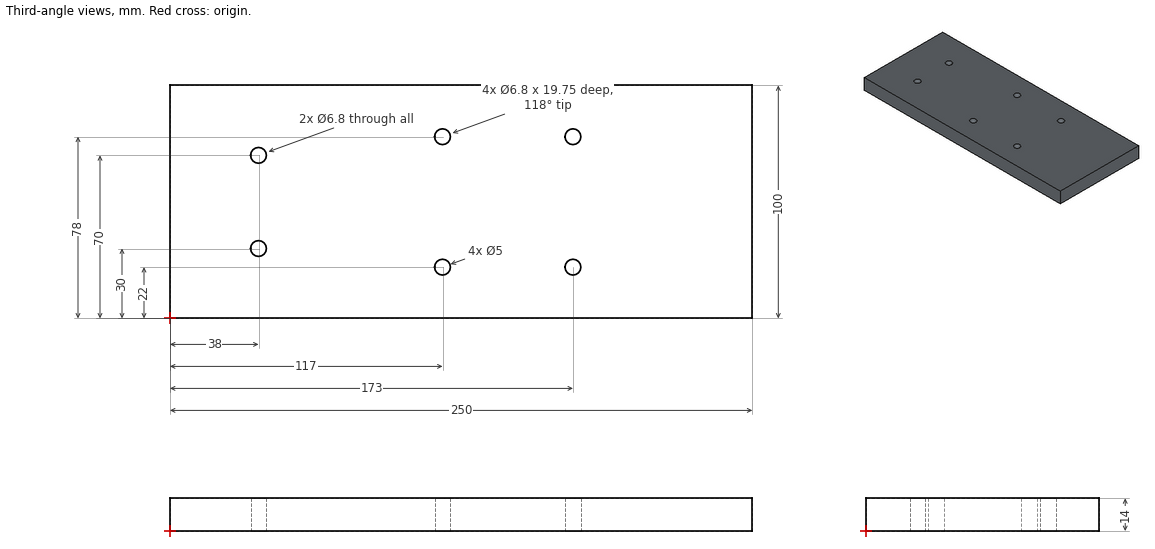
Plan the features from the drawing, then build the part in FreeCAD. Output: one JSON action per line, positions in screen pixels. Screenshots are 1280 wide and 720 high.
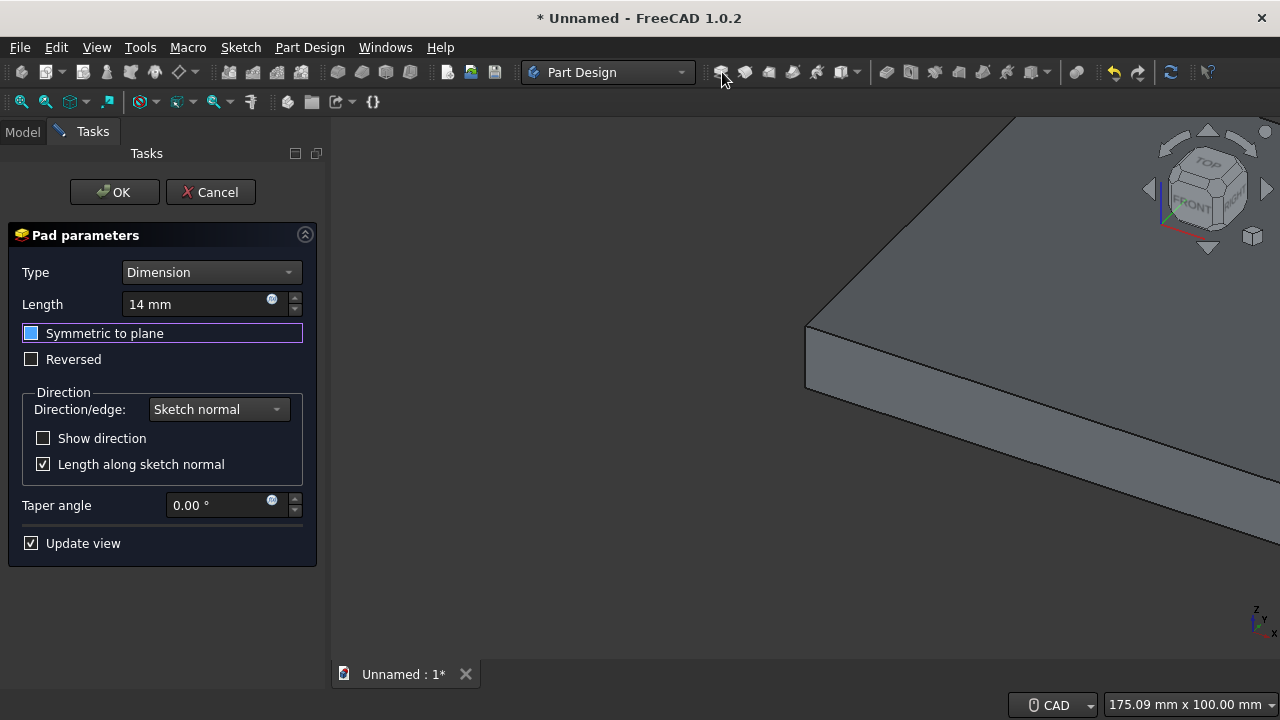
{"action": "left_click", "coordinate": [115, 192]}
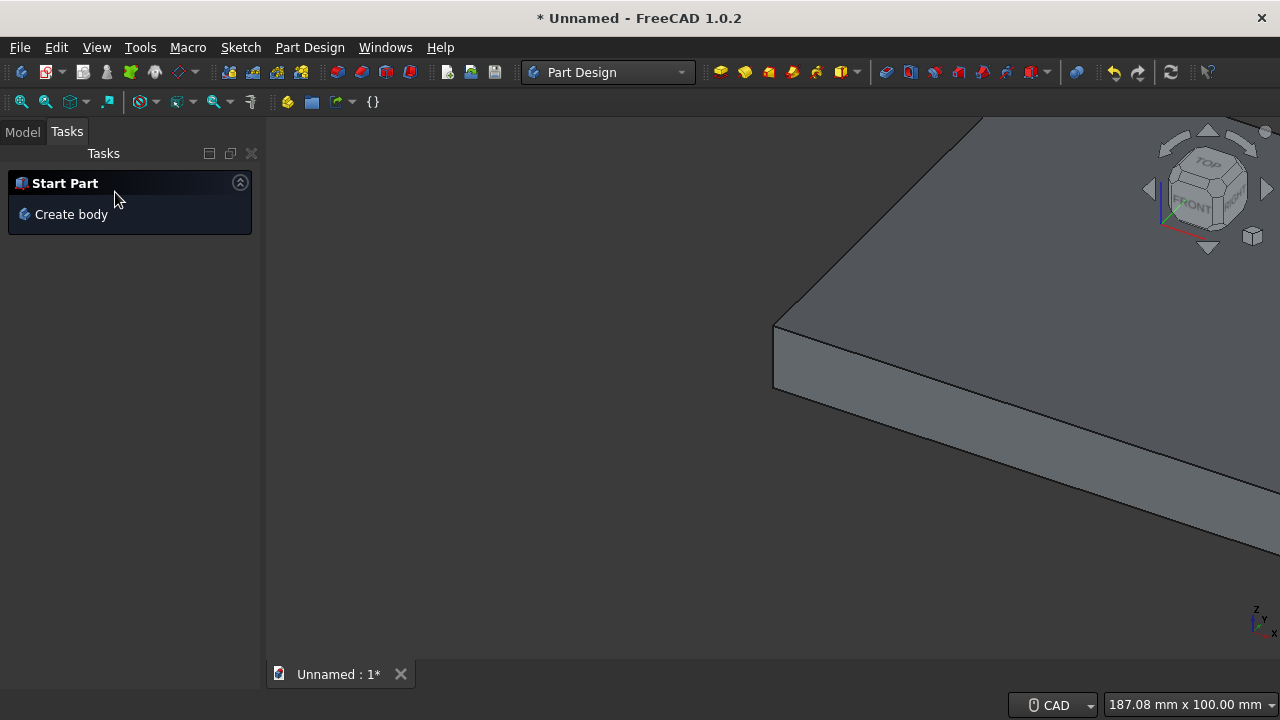
{"action": "left_click", "coordinate": [22, 102]}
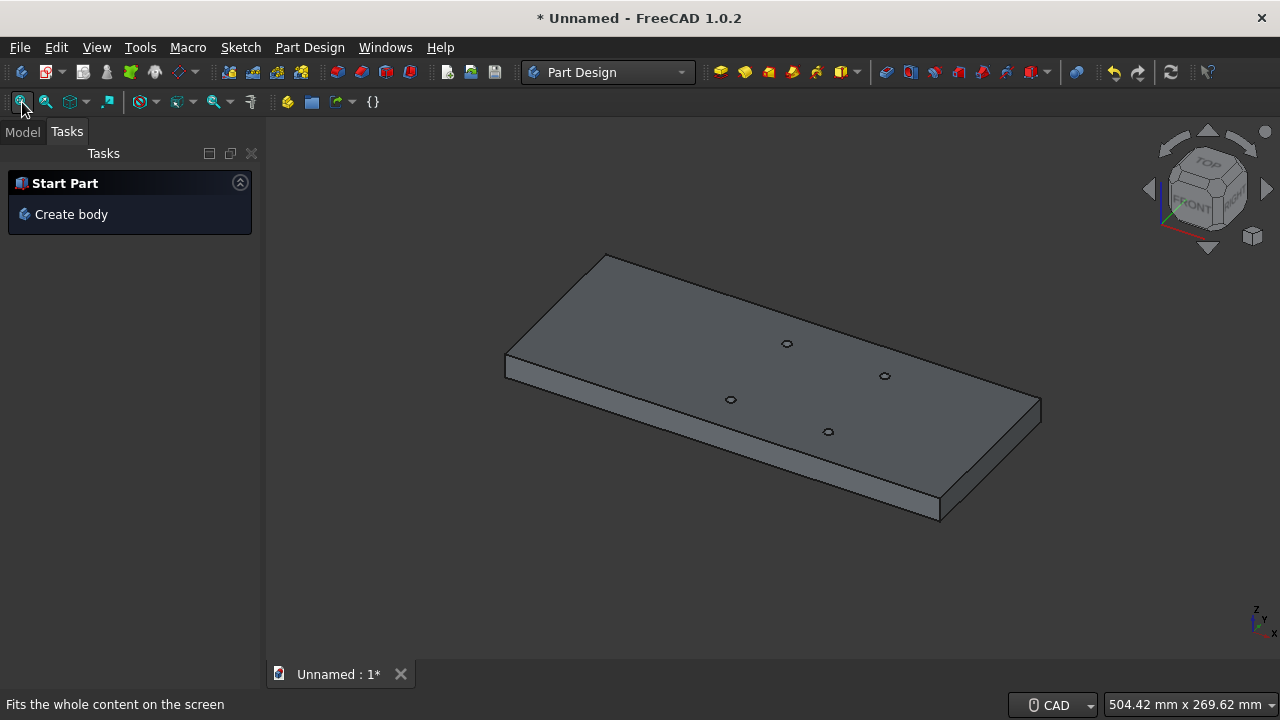
{"action": "left_click", "coordinate": [649, 334]}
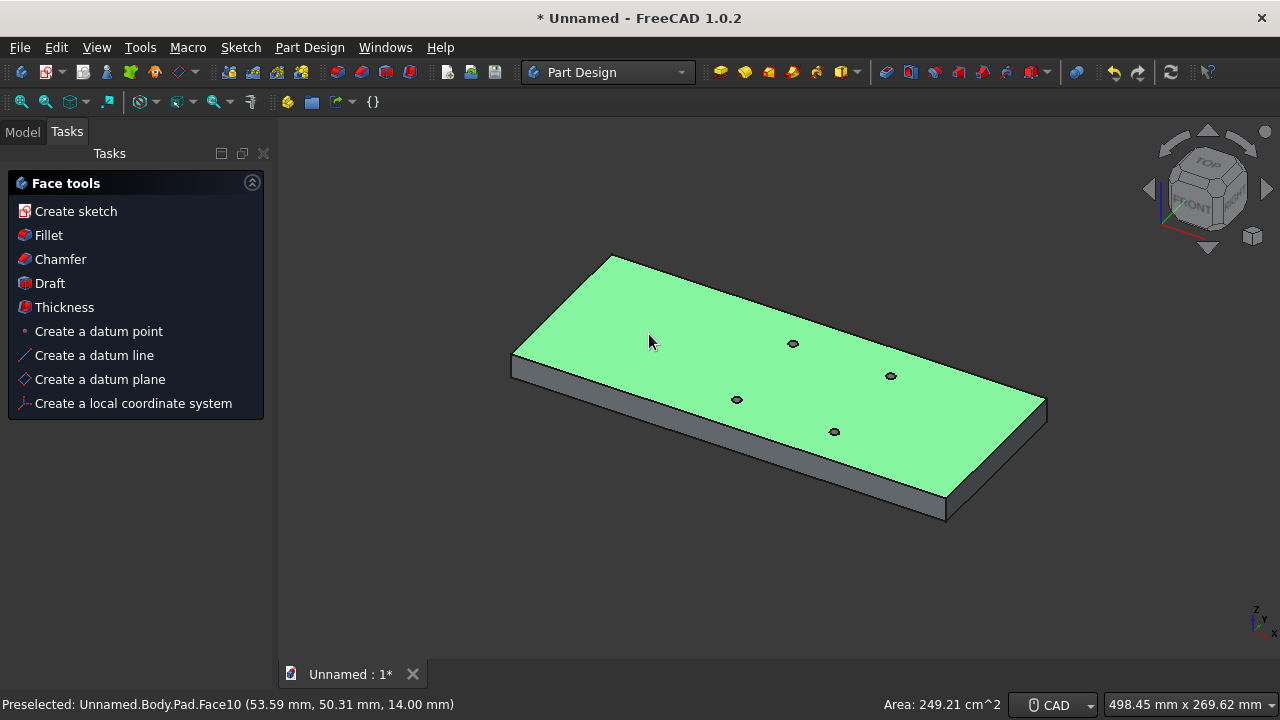
{"action": "left_click", "coordinate": [46, 72]}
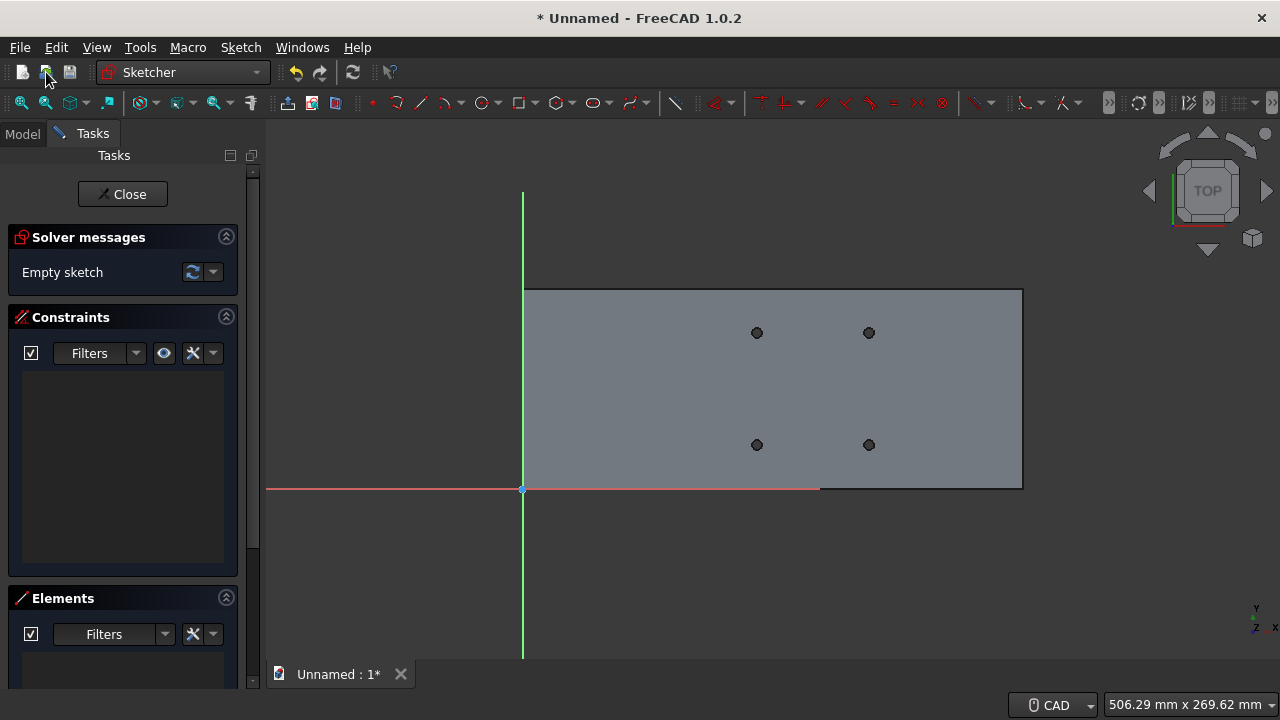
{"action": "scroll", "coordinate": [876, 389], "scroll_direction": "up", "scroll_amount": 5}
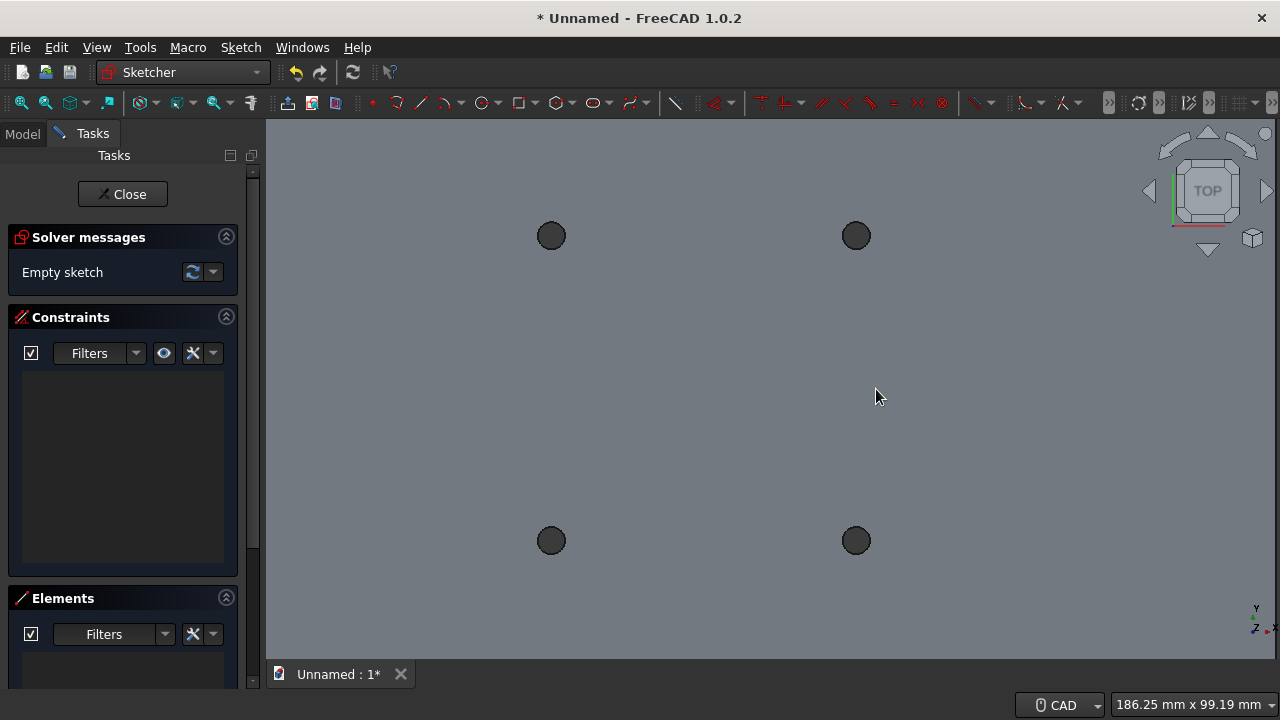
{"action": "left_click", "coordinate": [482, 104]}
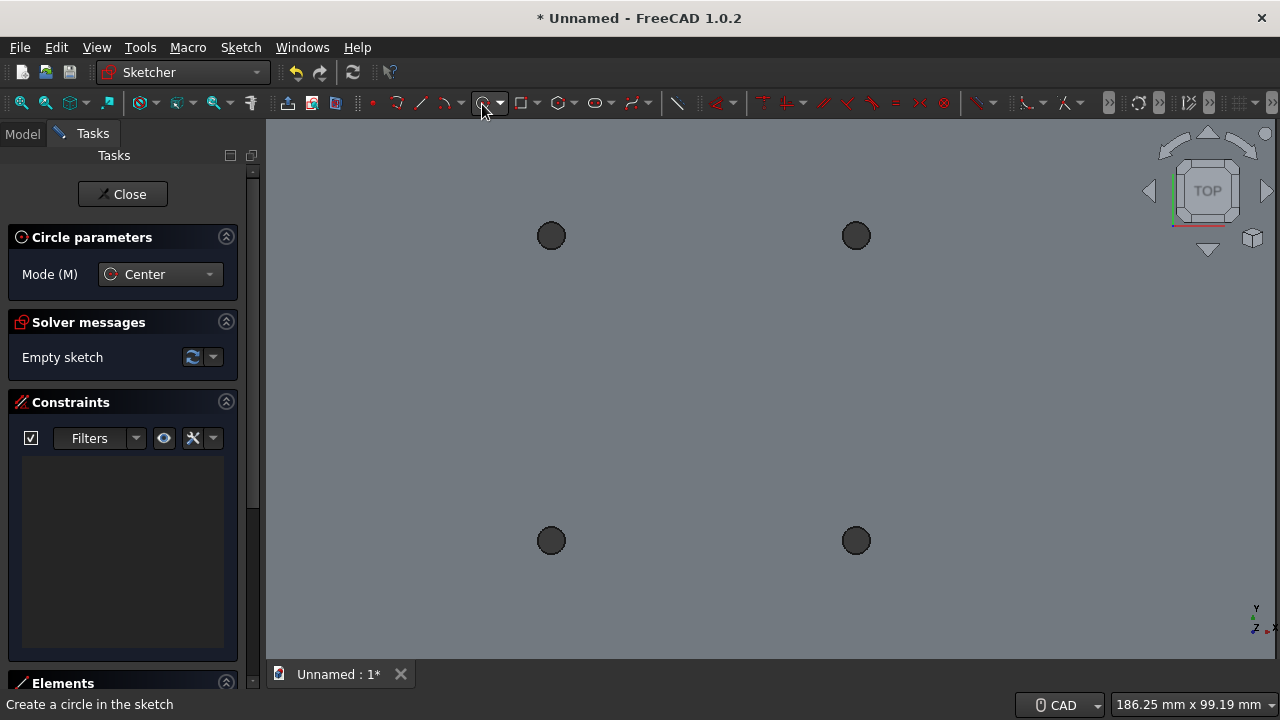
{"action": "scroll", "coordinate": [551, 236], "scroll_direction": "up", "scroll_amount": 2}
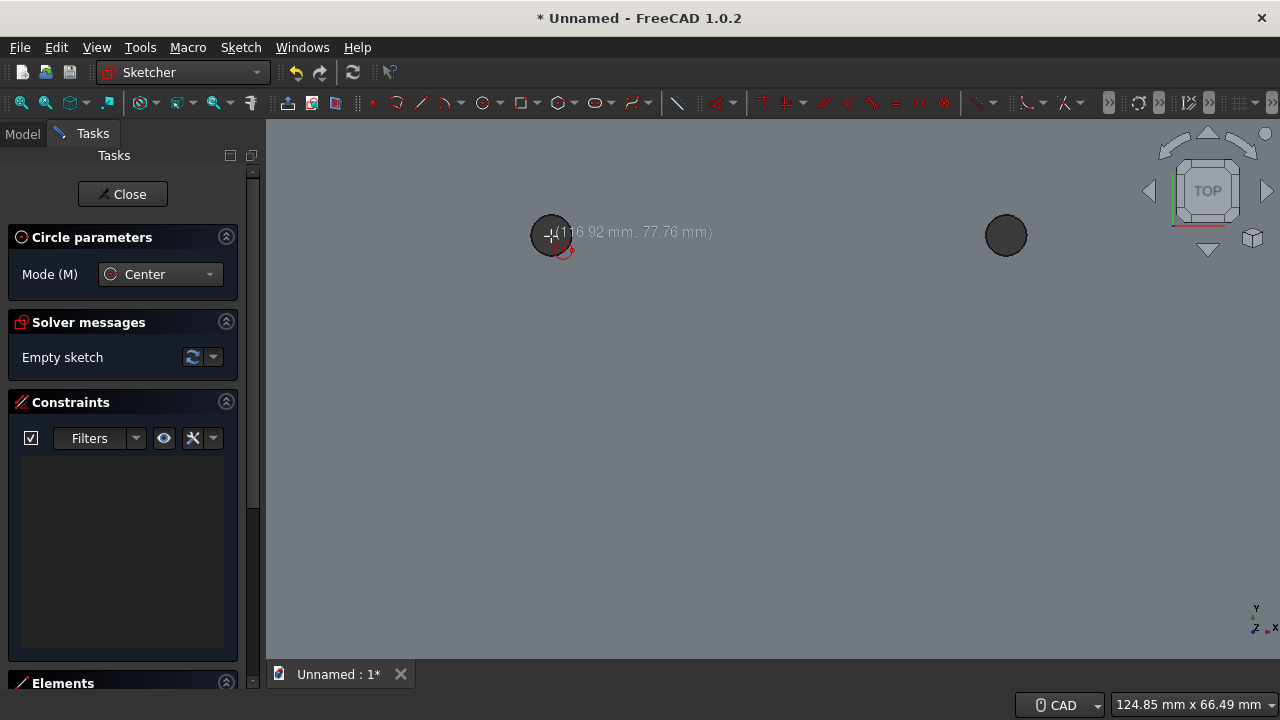
{"action": "left_click", "coordinate": [552, 235]}
{"action": "left_click", "coordinate": [571, 216]}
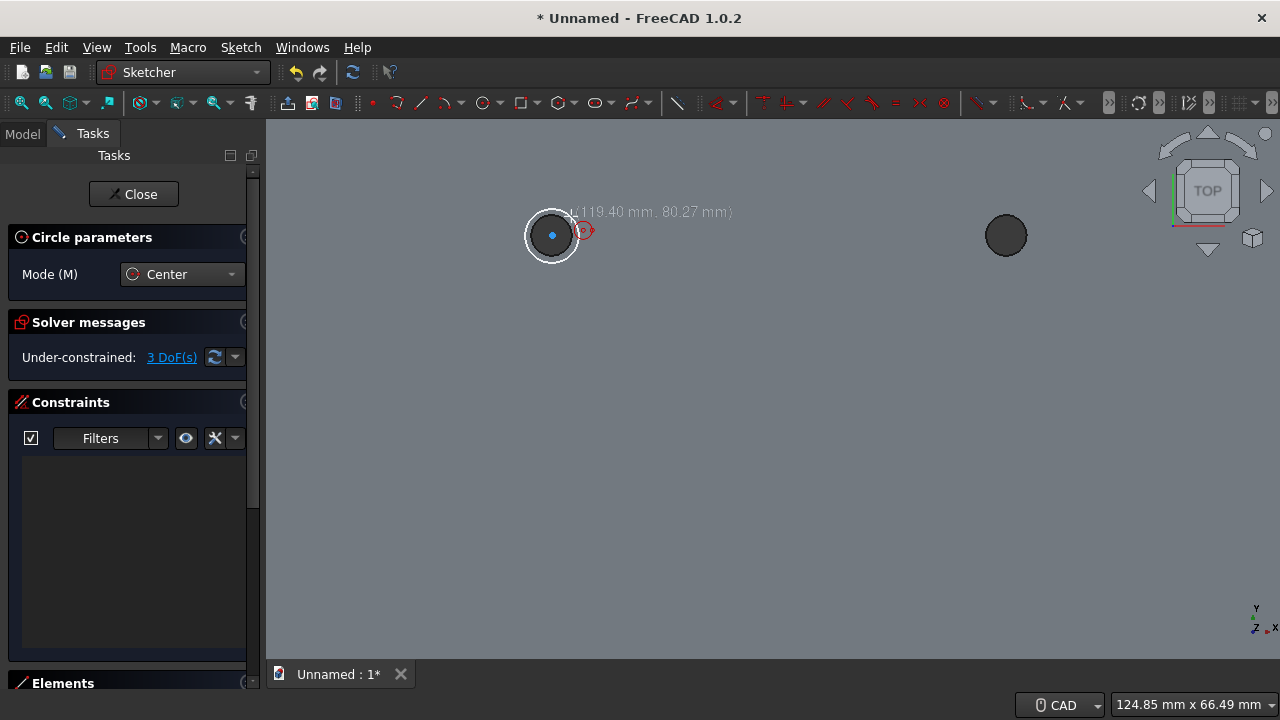
{"action": "left_click", "coordinate": [1006, 235]}
{"action": "left_click", "coordinate": [1026, 216]}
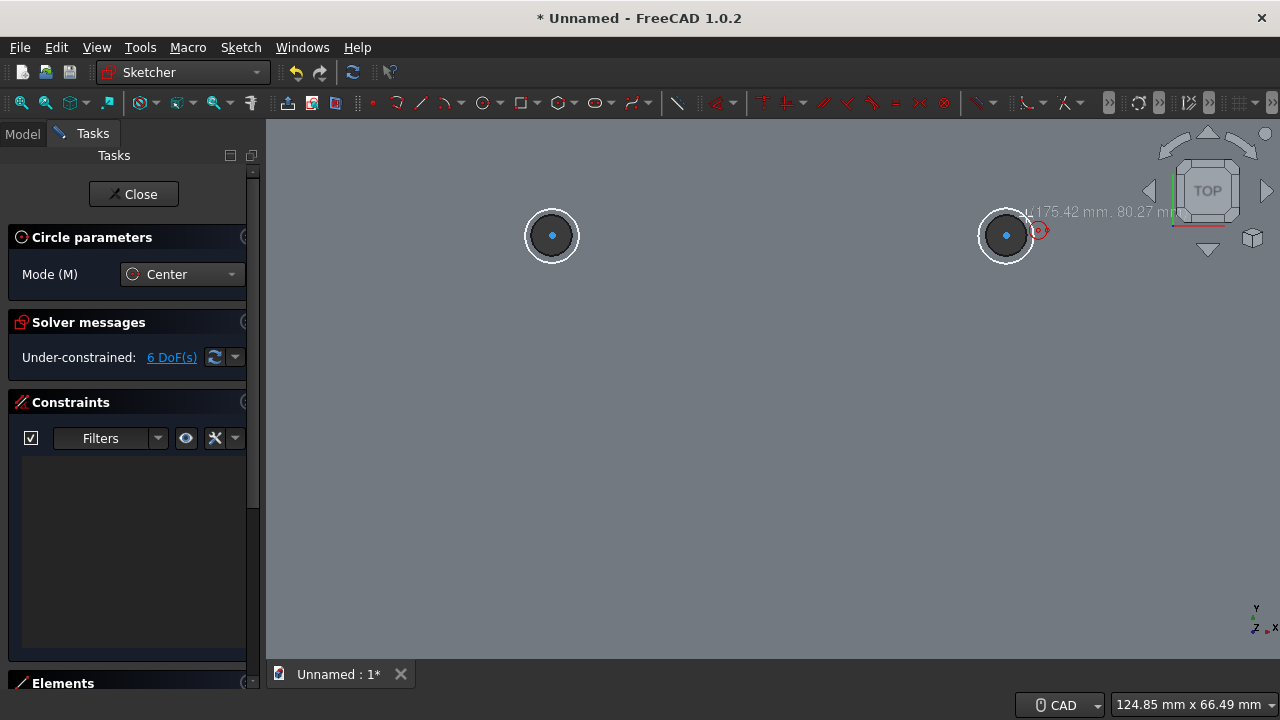
{"action": "scroll", "coordinate": [553, 239], "scroll_direction": "down", "scroll_amount": 2}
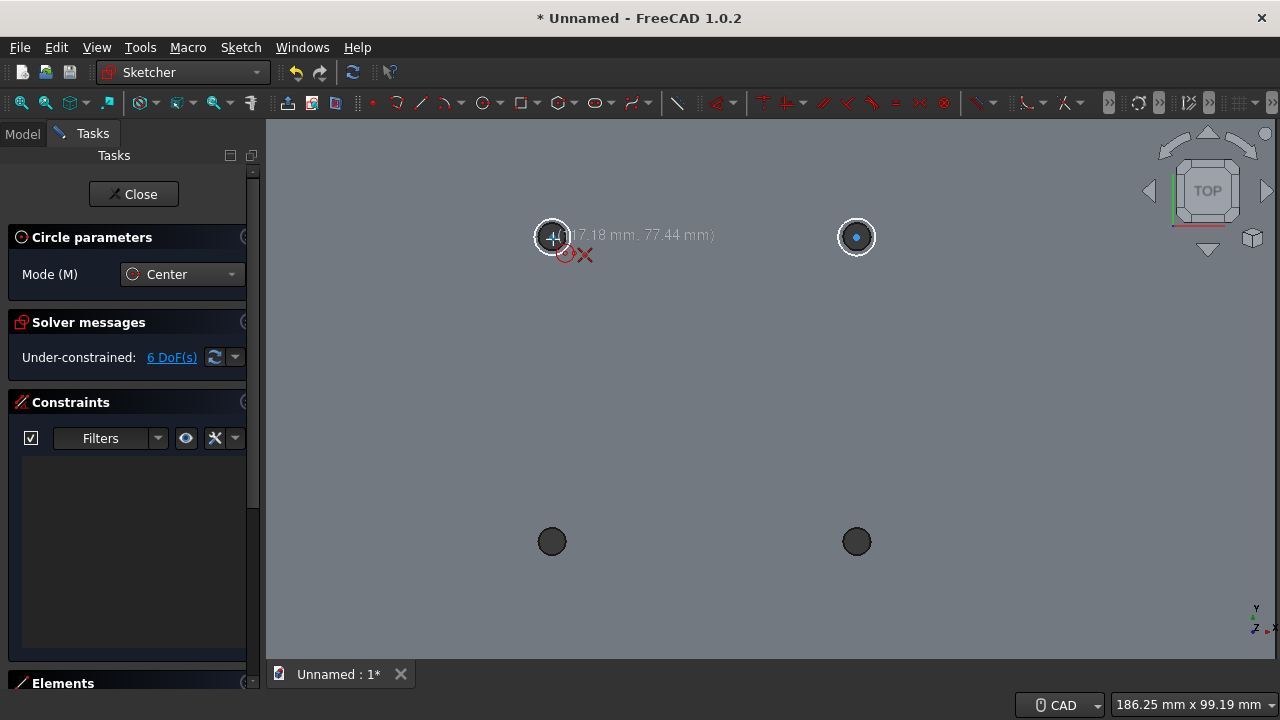
{"action": "scroll", "coordinate": [552, 542], "scroll_direction": "up", "scroll_amount": 2}